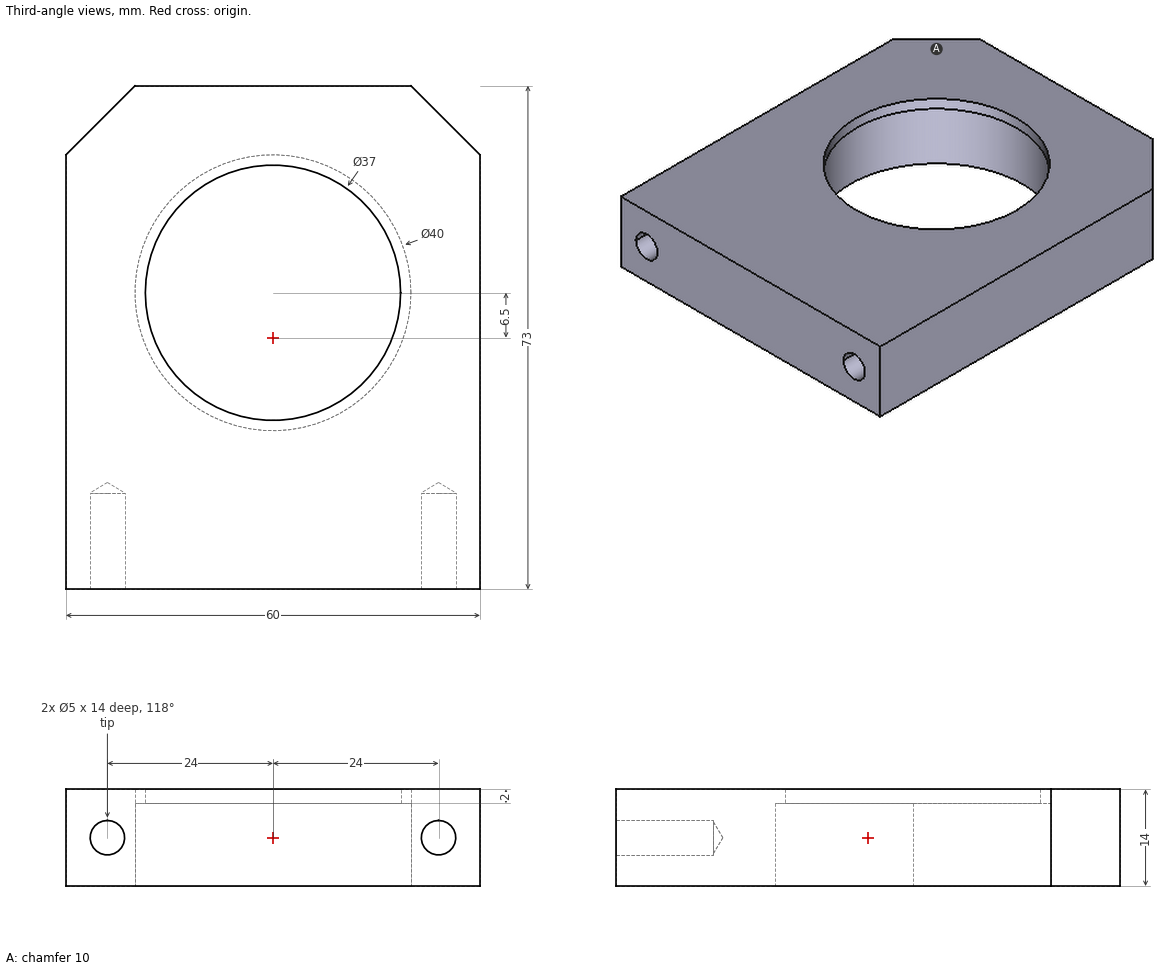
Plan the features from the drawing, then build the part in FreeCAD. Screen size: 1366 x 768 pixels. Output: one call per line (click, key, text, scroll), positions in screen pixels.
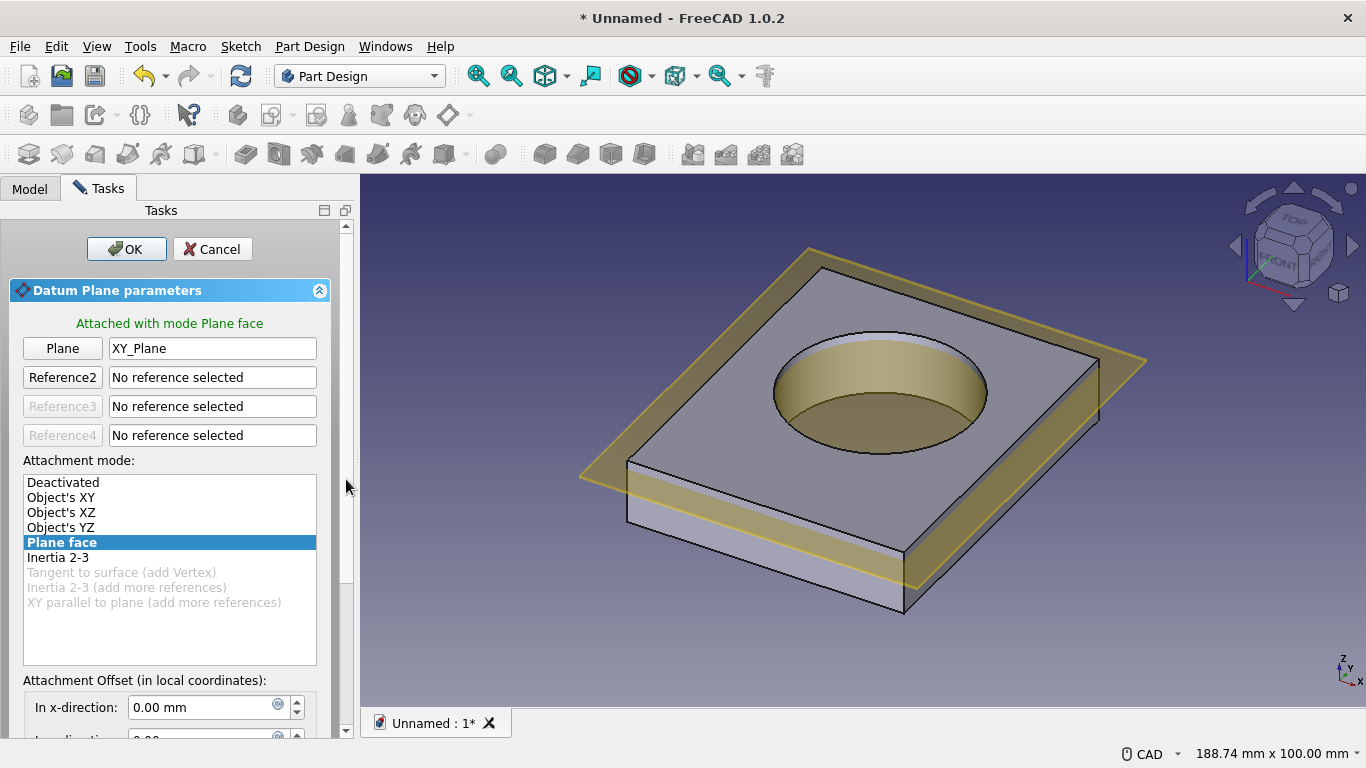
click(127, 249)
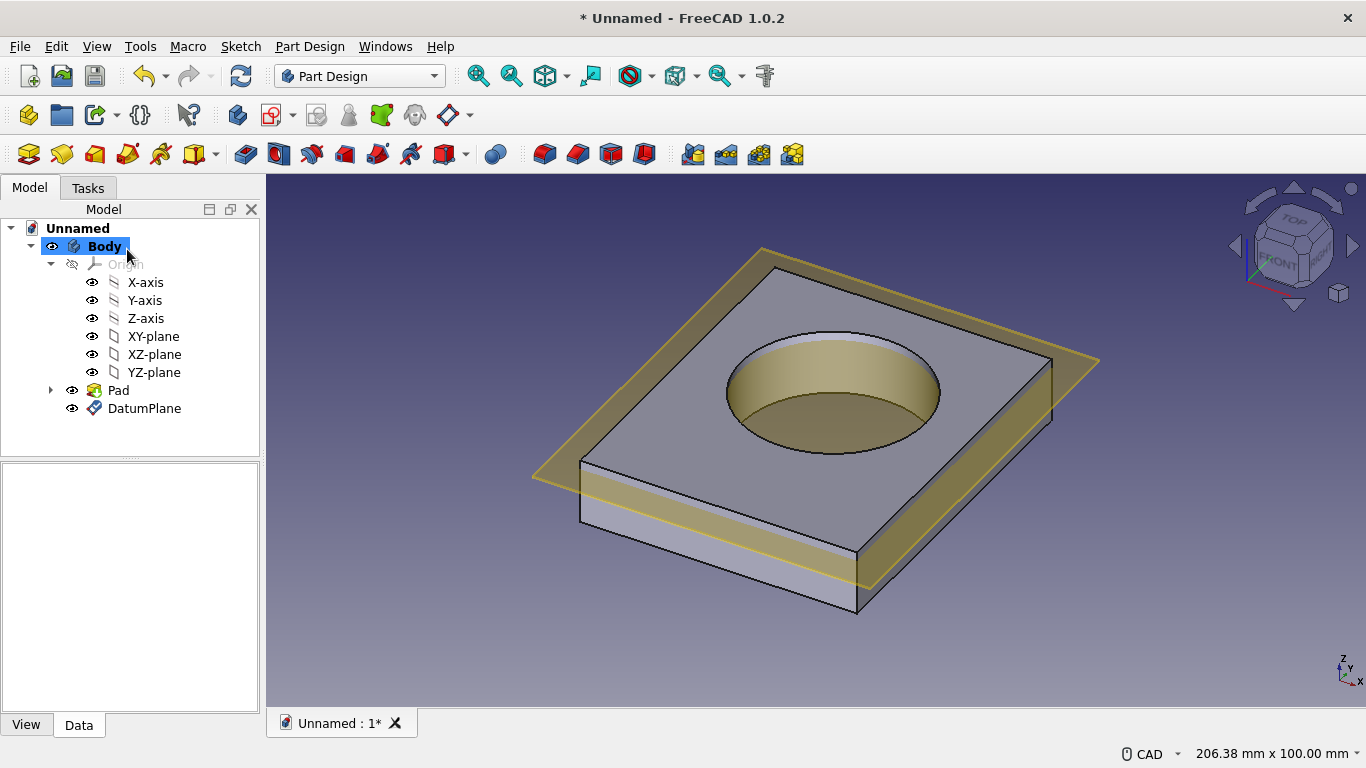
click(117, 408)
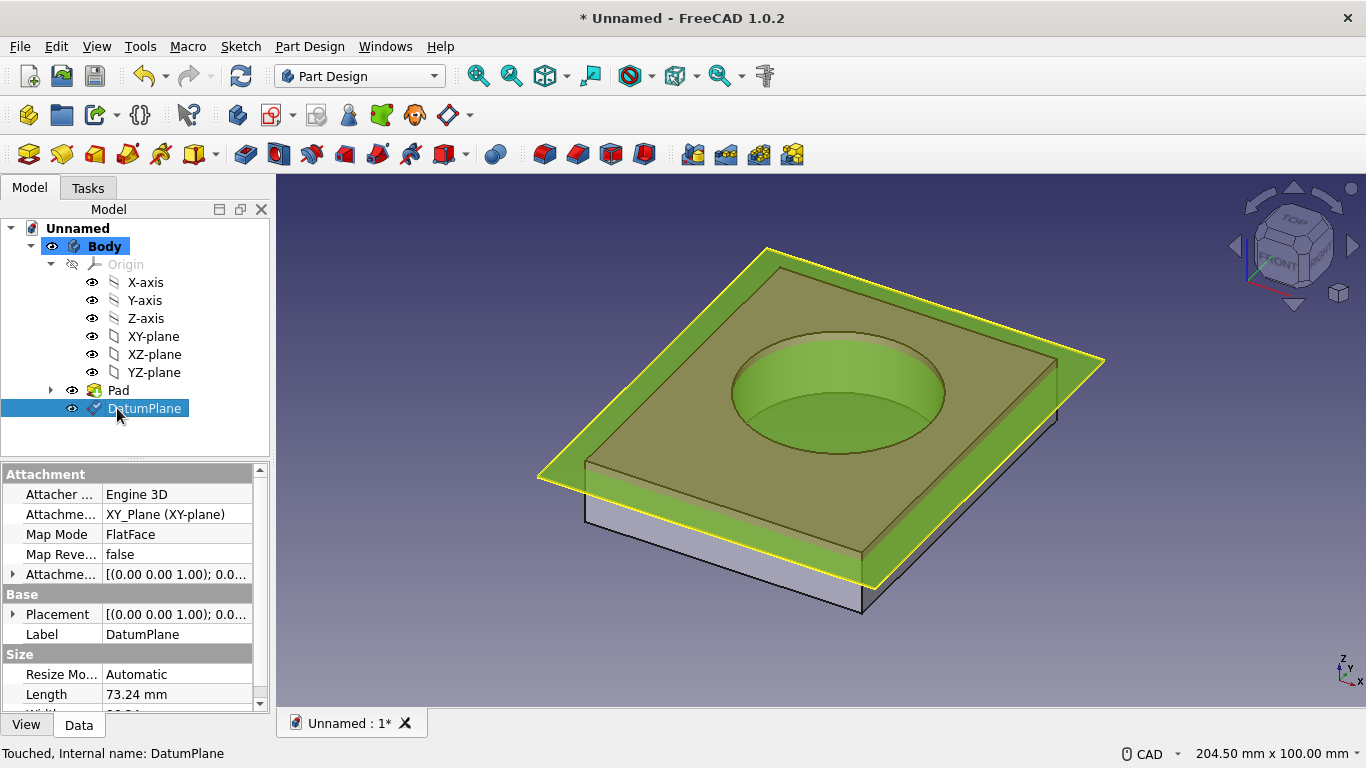
click(270, 116)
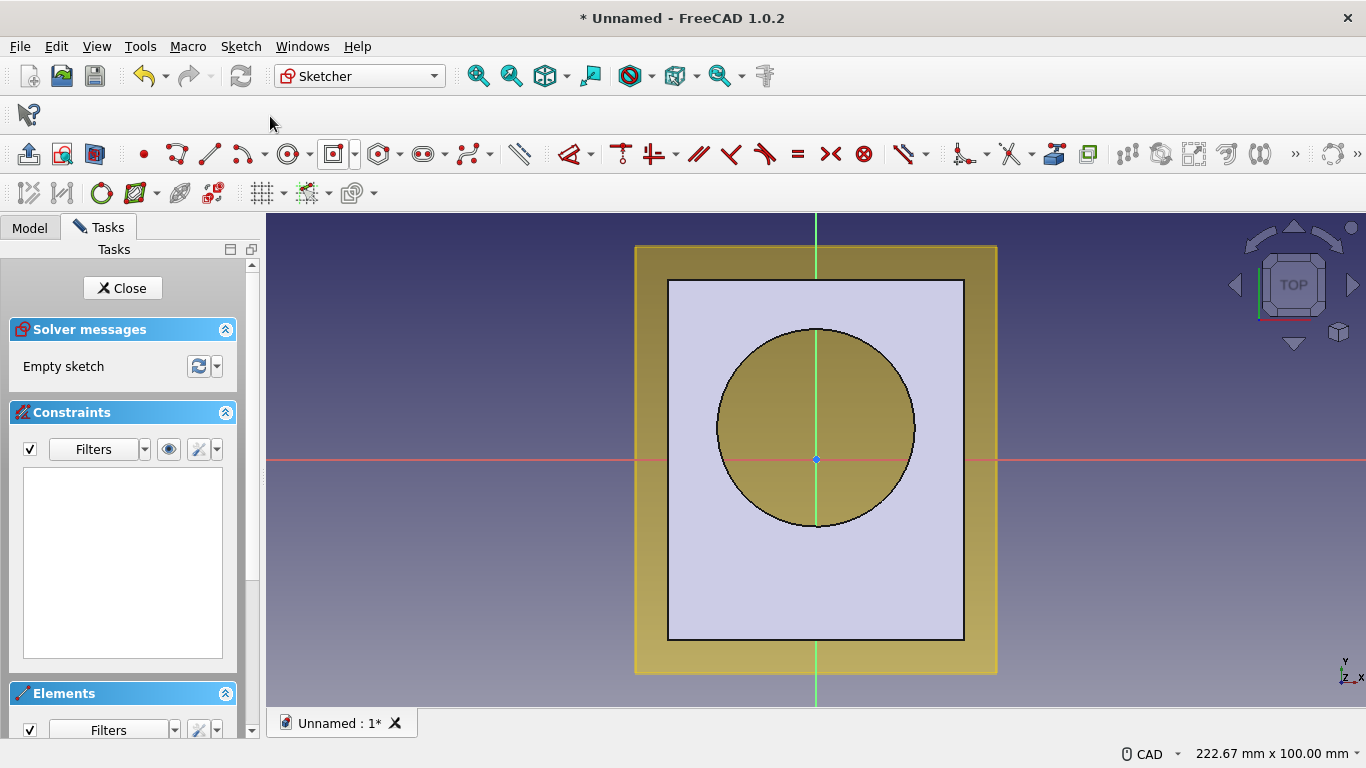
click(95, 154)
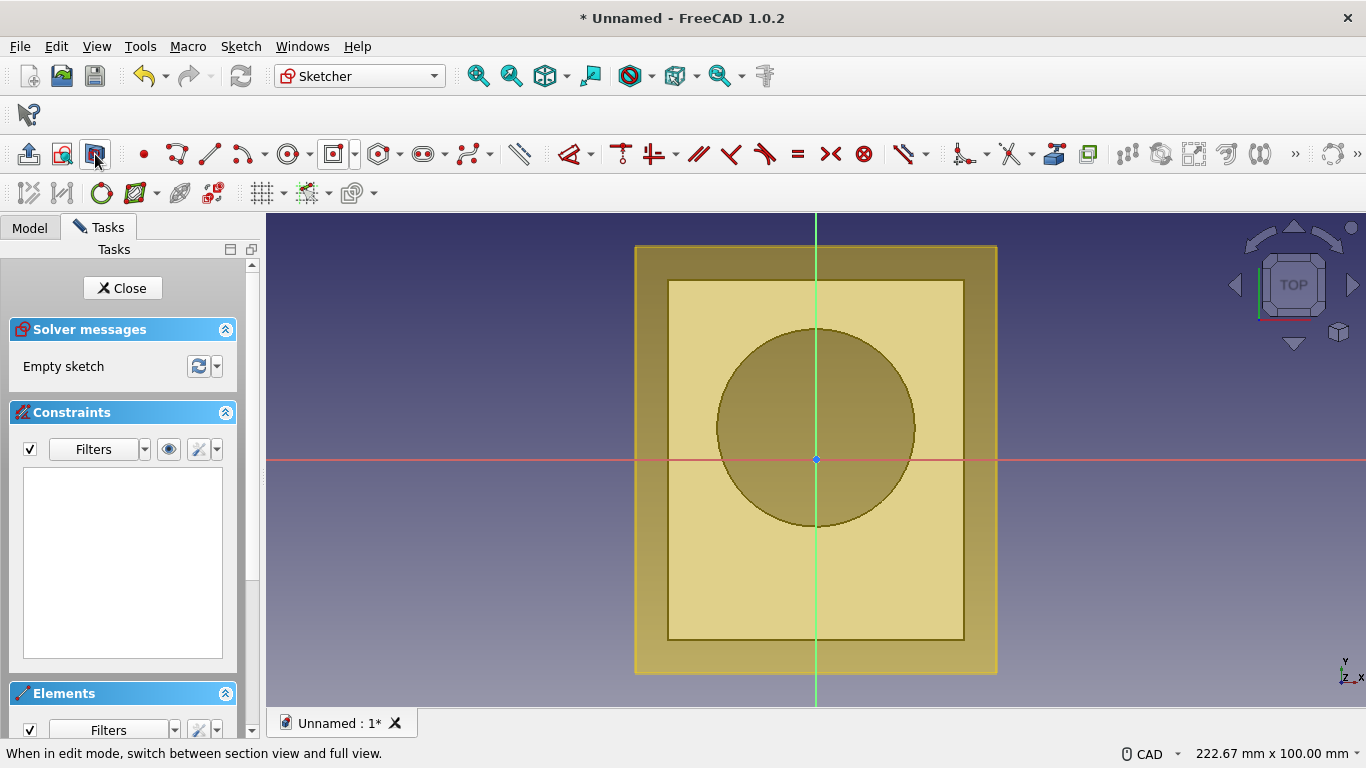
scroll(955, 363, up, 2)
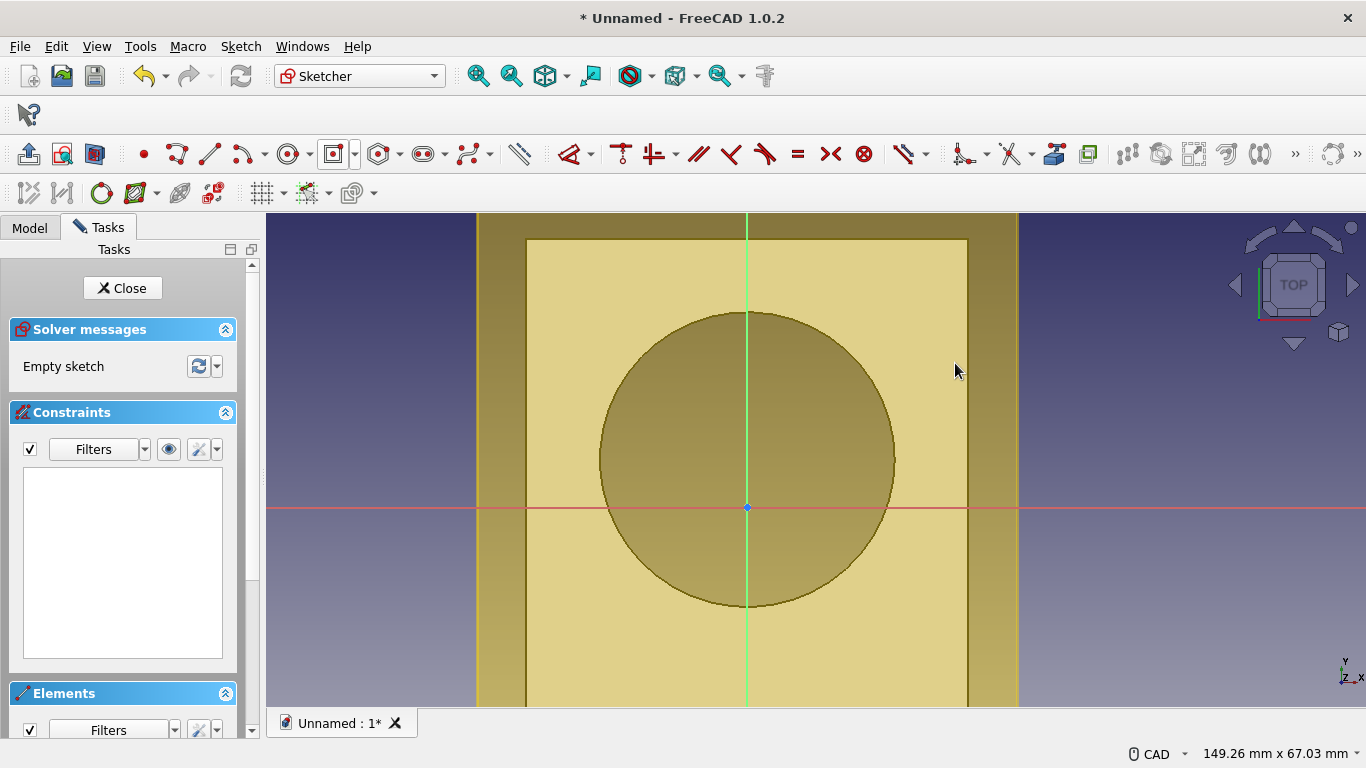
click(288, 154)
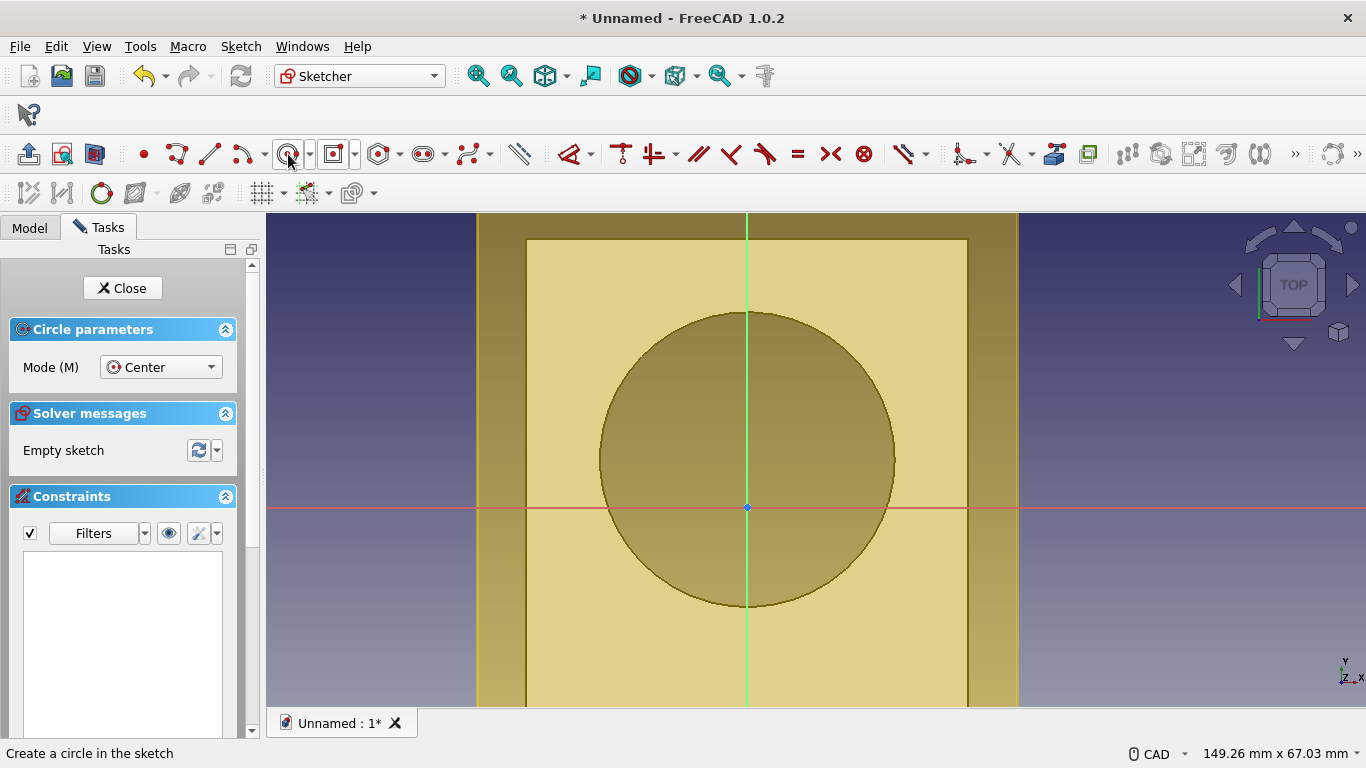
click(747, 460)
move(852, 355)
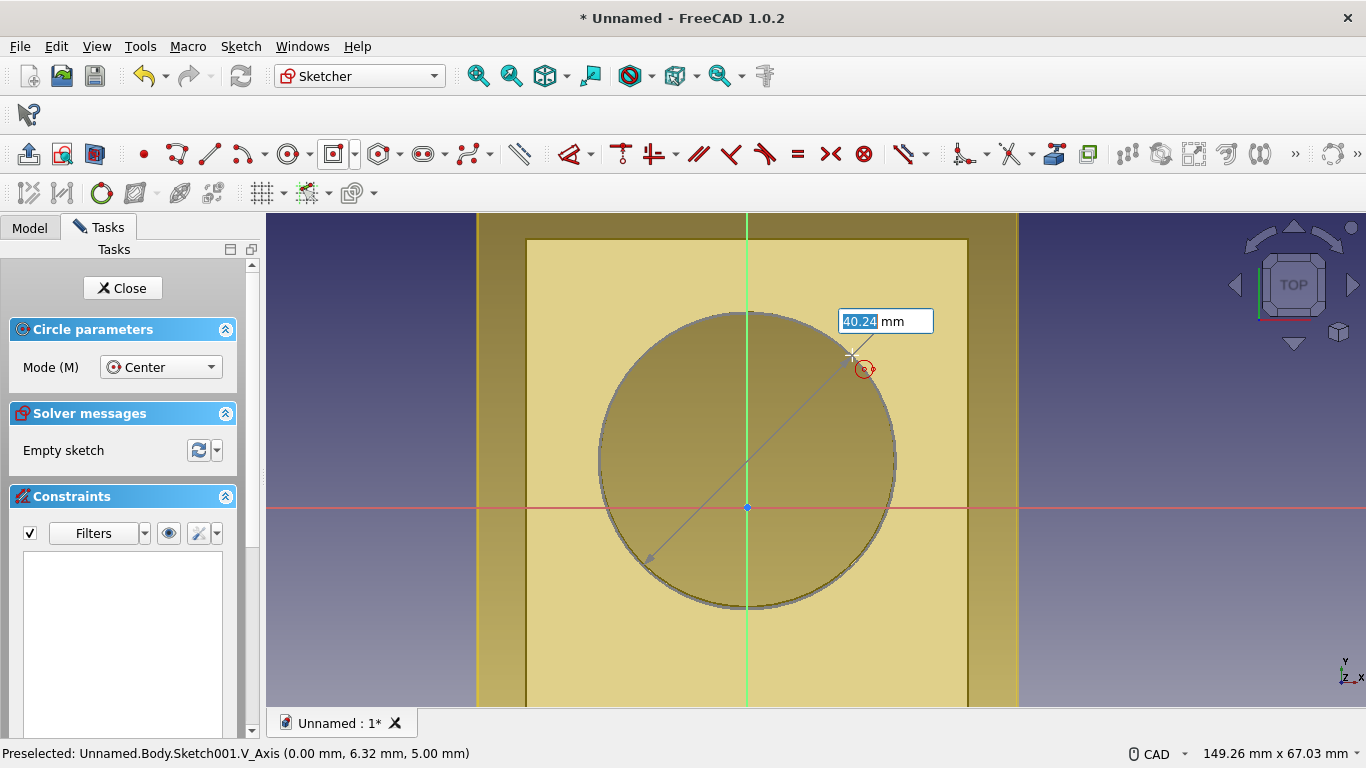
text(40)
key(Return)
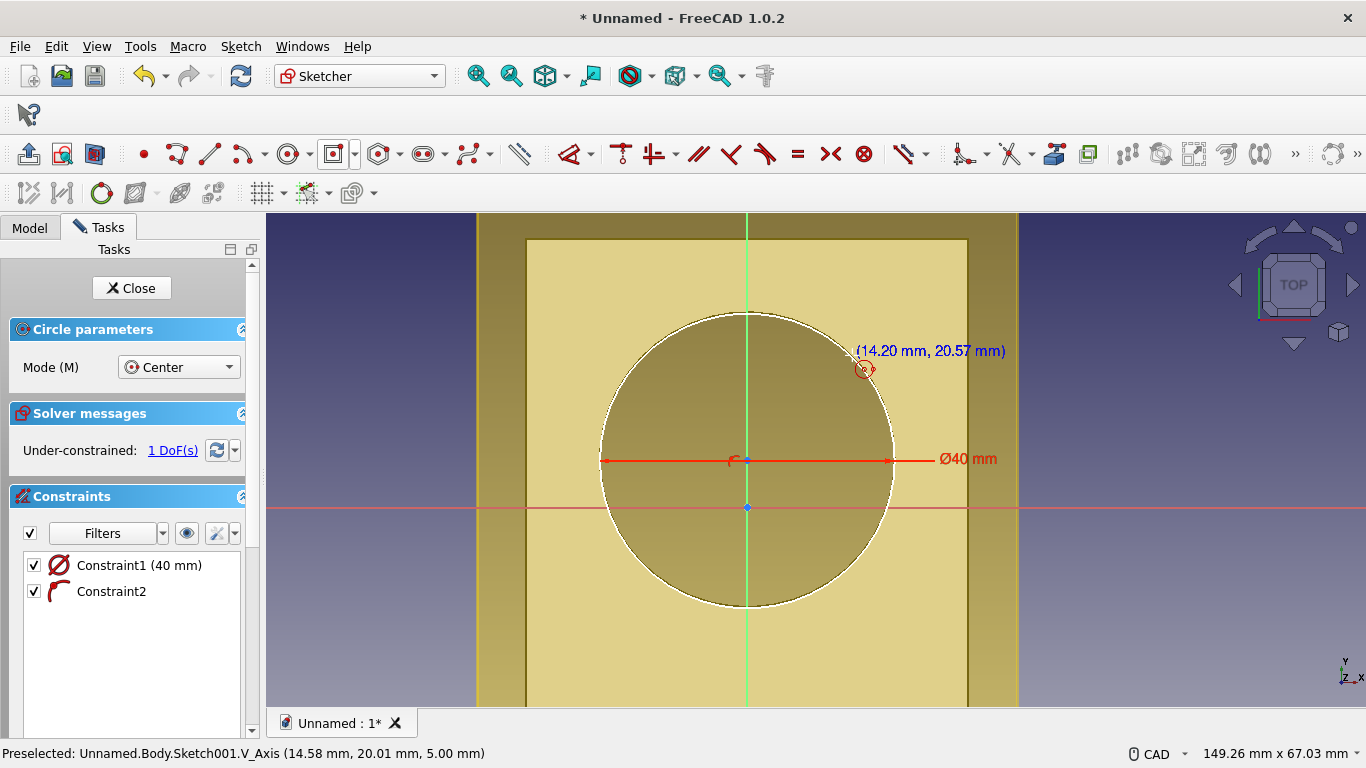
click(747, 461)